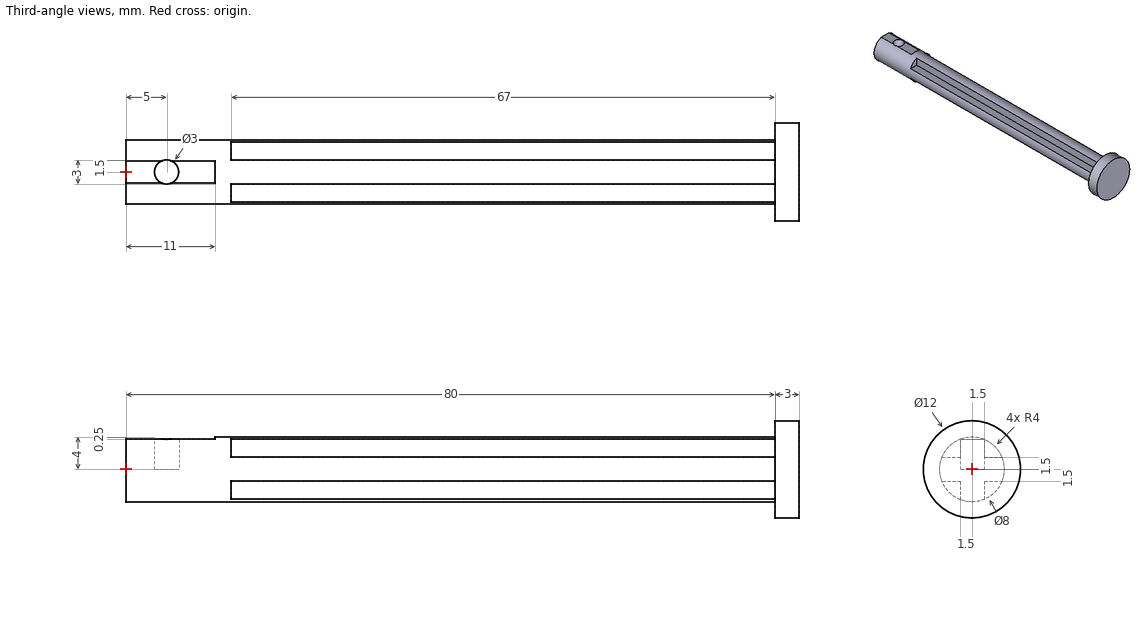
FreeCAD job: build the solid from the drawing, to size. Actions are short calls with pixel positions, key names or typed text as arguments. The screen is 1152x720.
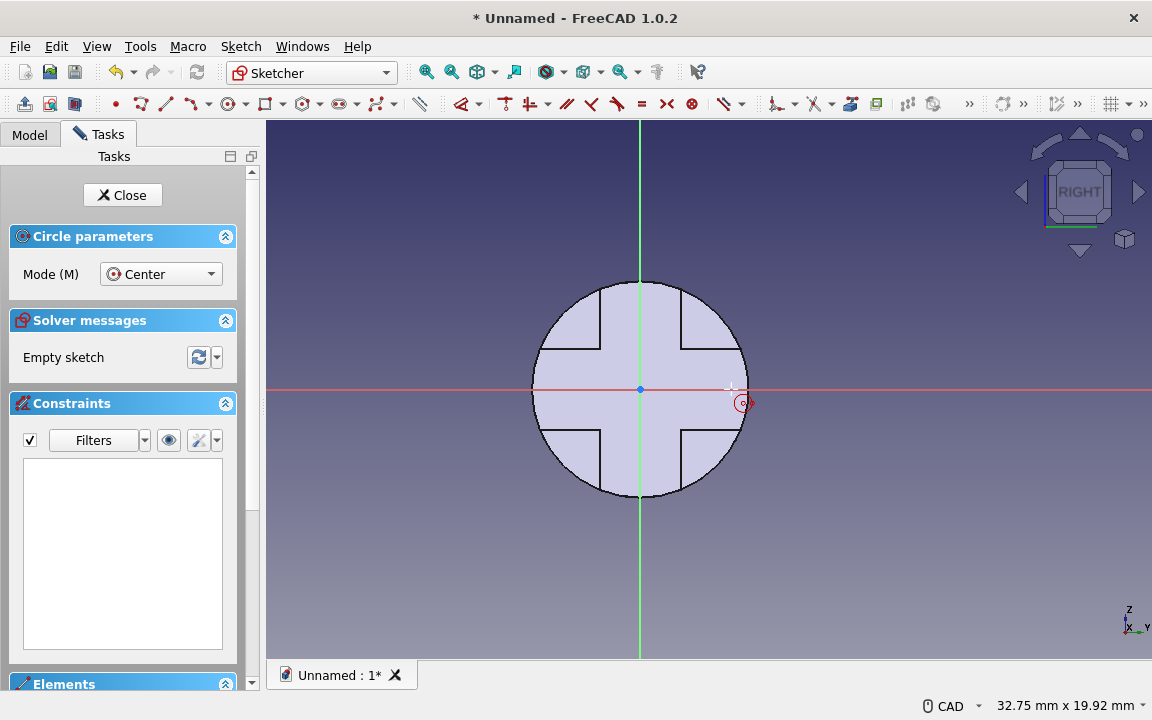
click(640, 389)
move(755, 275)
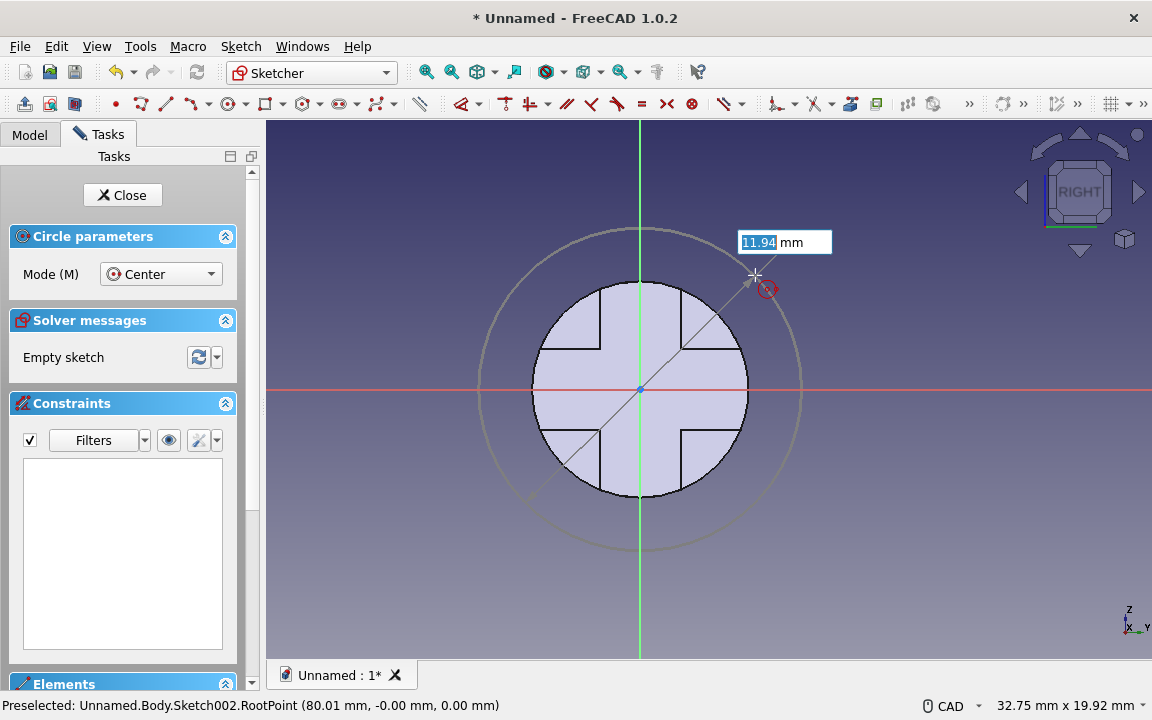
text(12)
key(Return)
key(Escape)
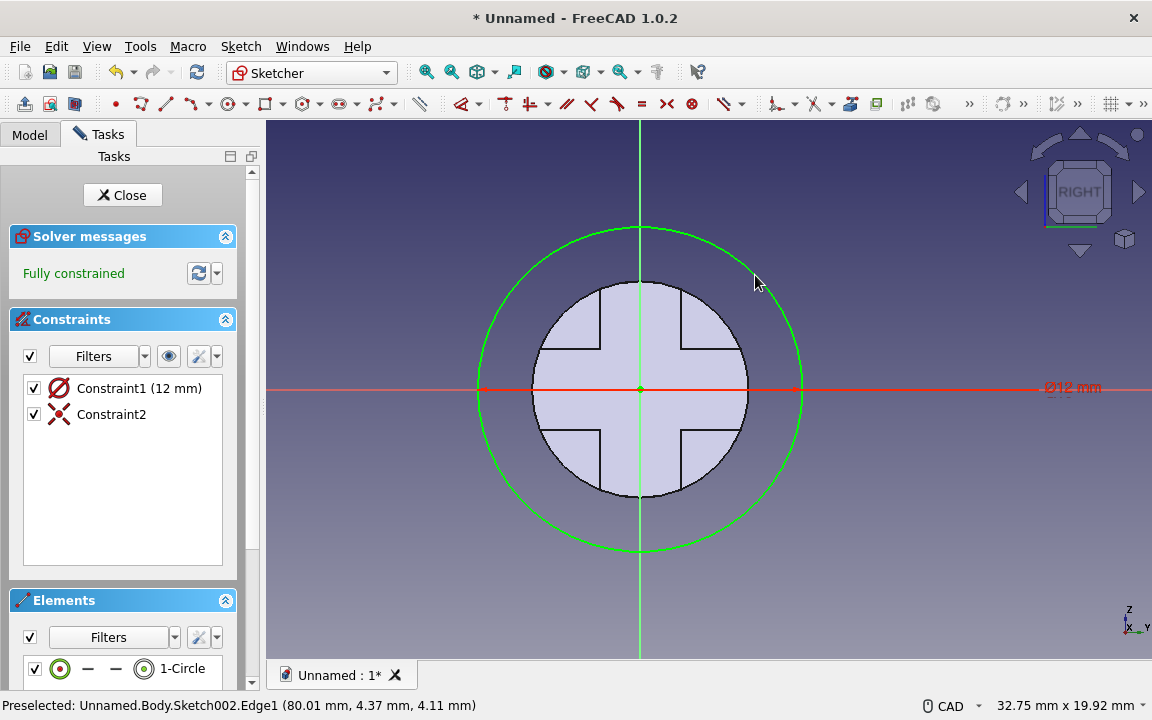
click(123, 195)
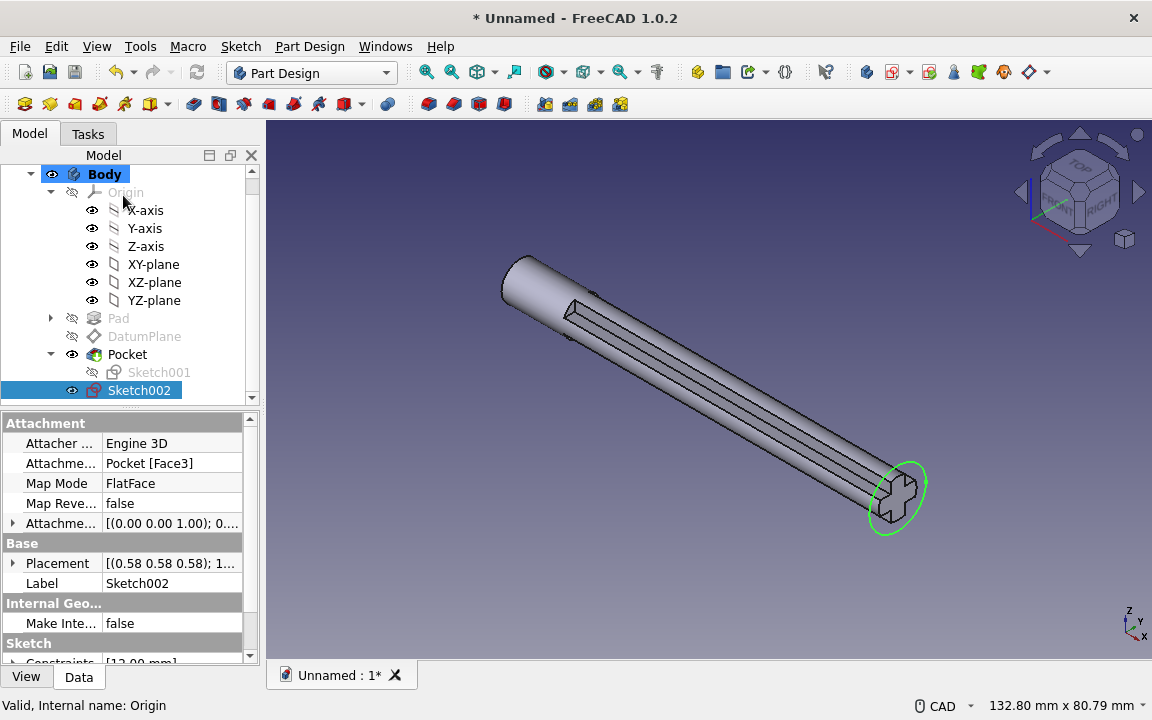
click(25, 104)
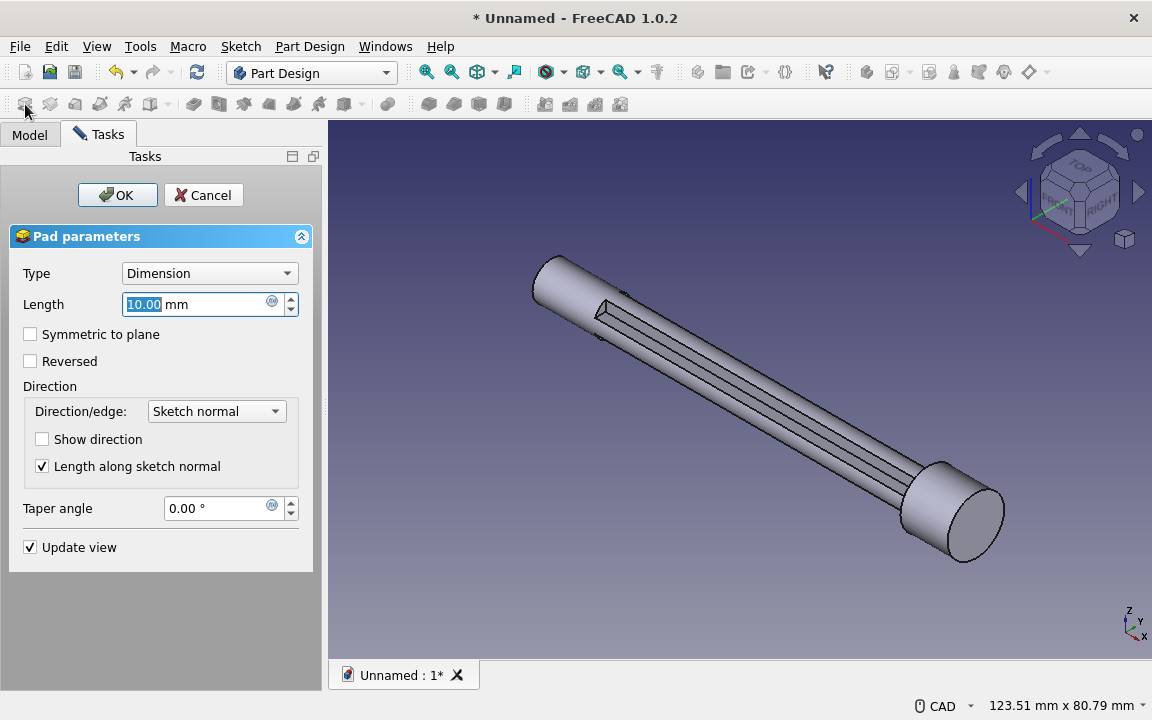
text(3)
key(Tab)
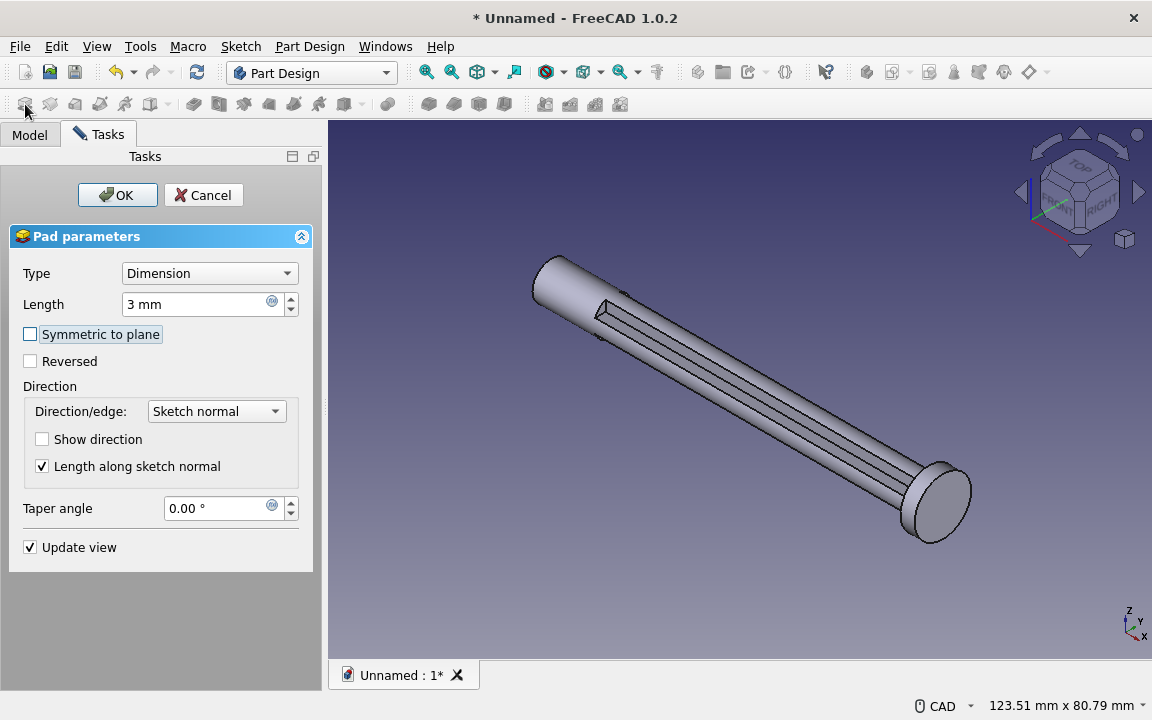
click(118, 195)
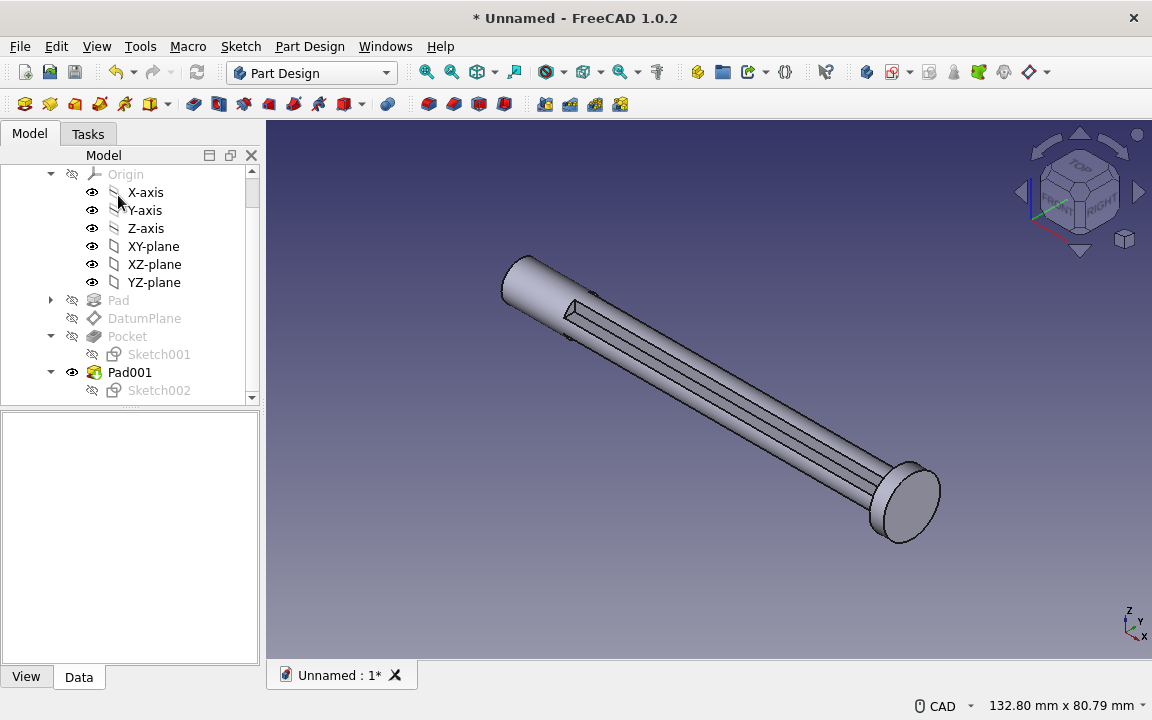
click(137, 246)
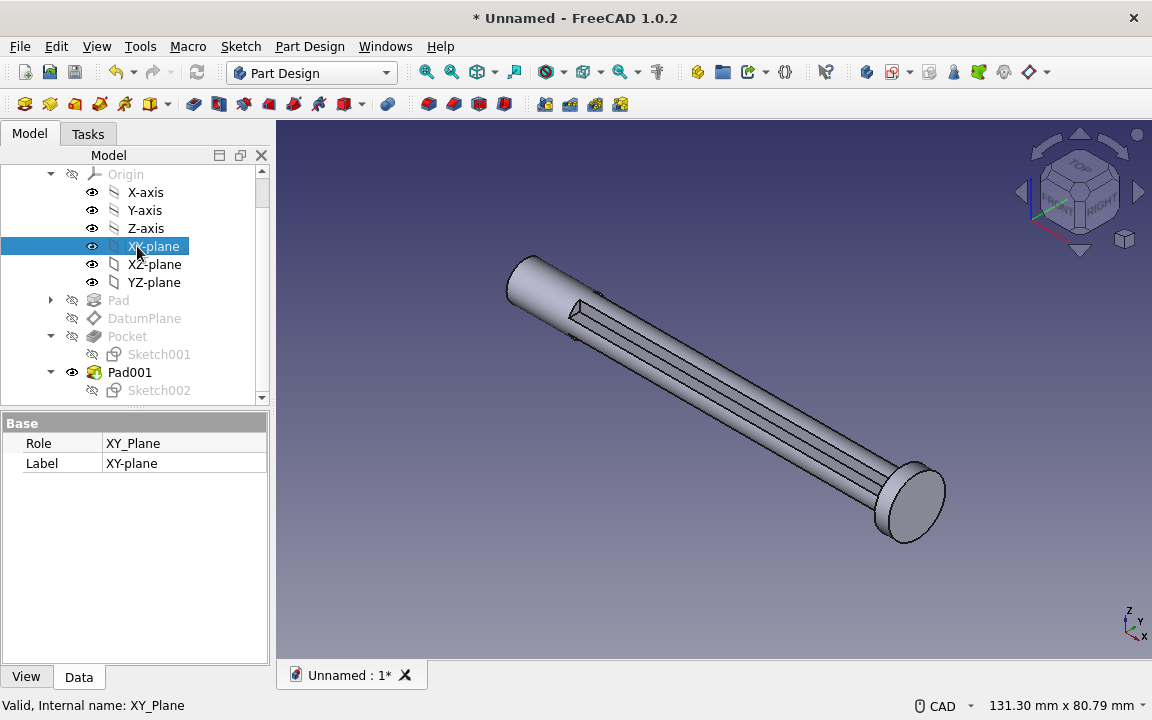
click(1028, 72)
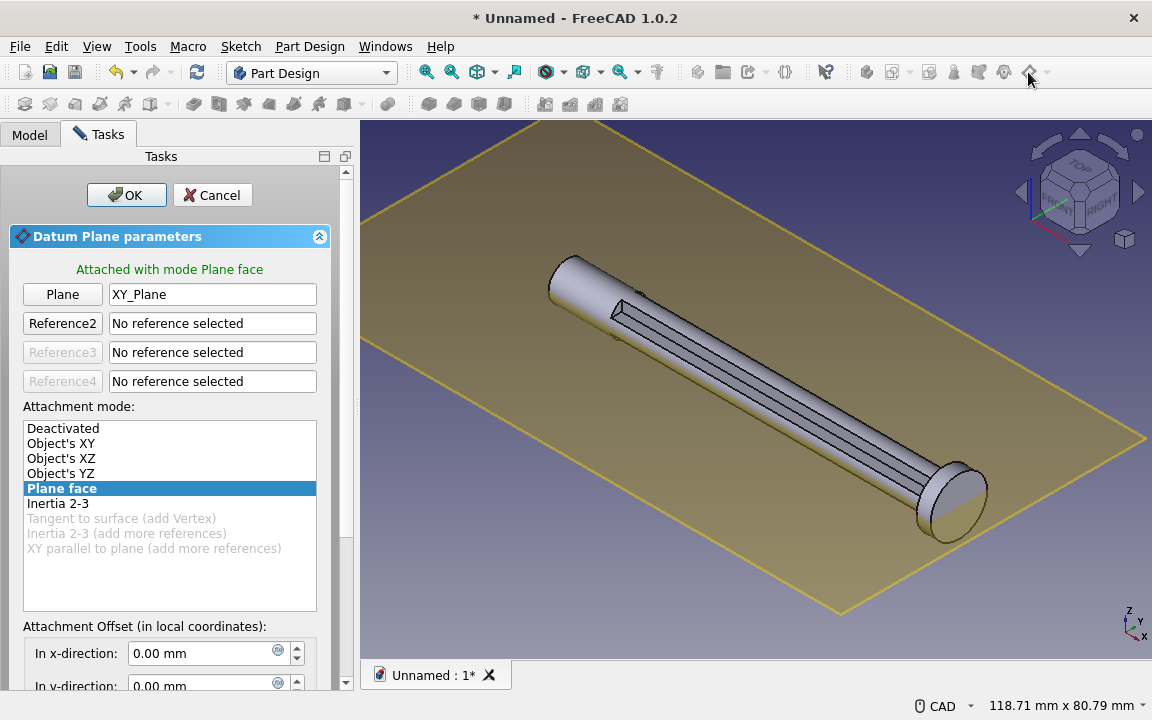
scroll(346, 428, down, 2)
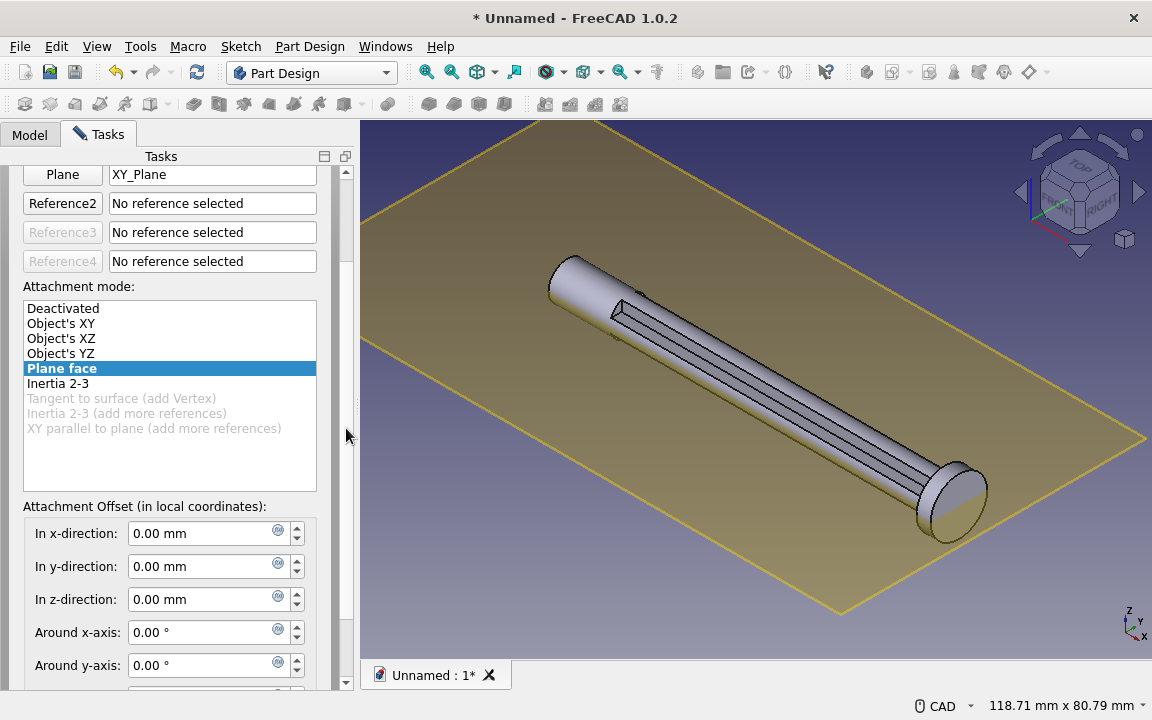
triple_click(210, 600)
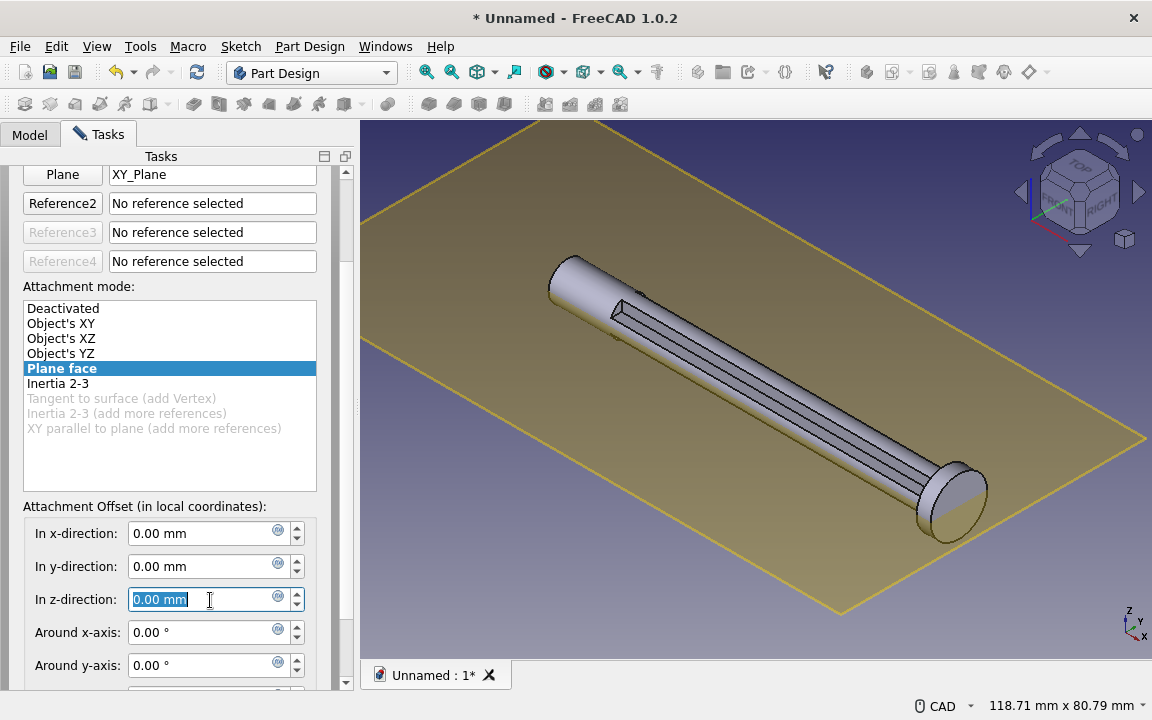
text(4)
key(Tab)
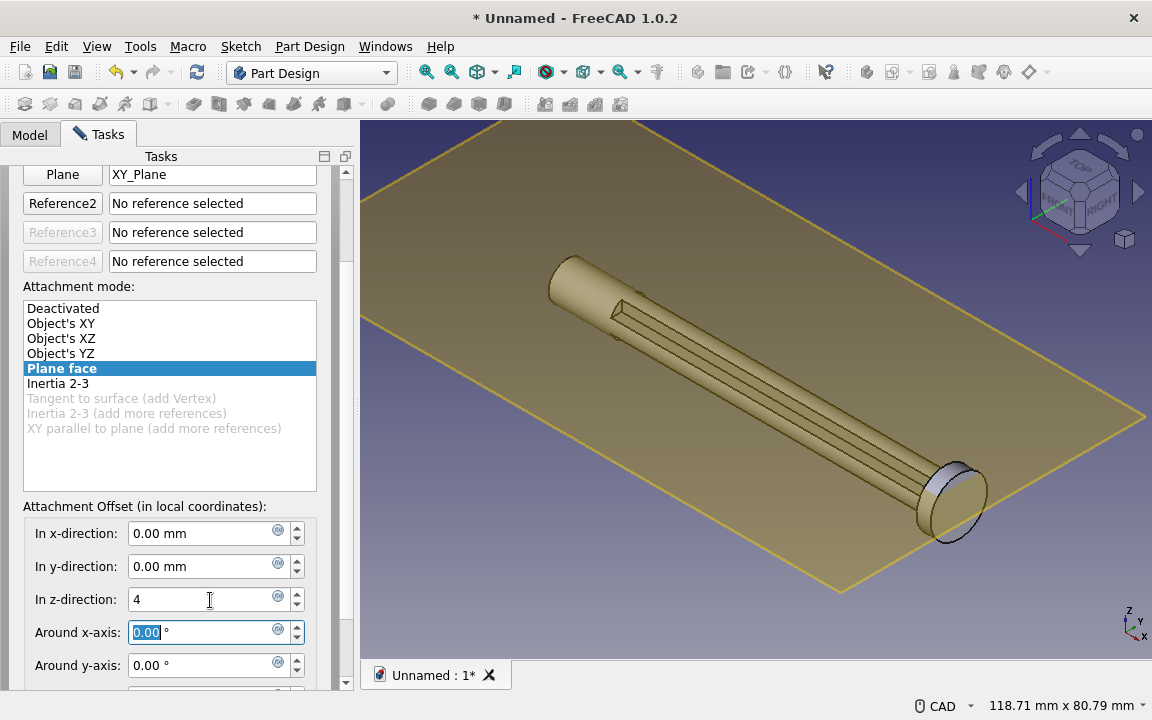
scroll(346, 428, up, 3)